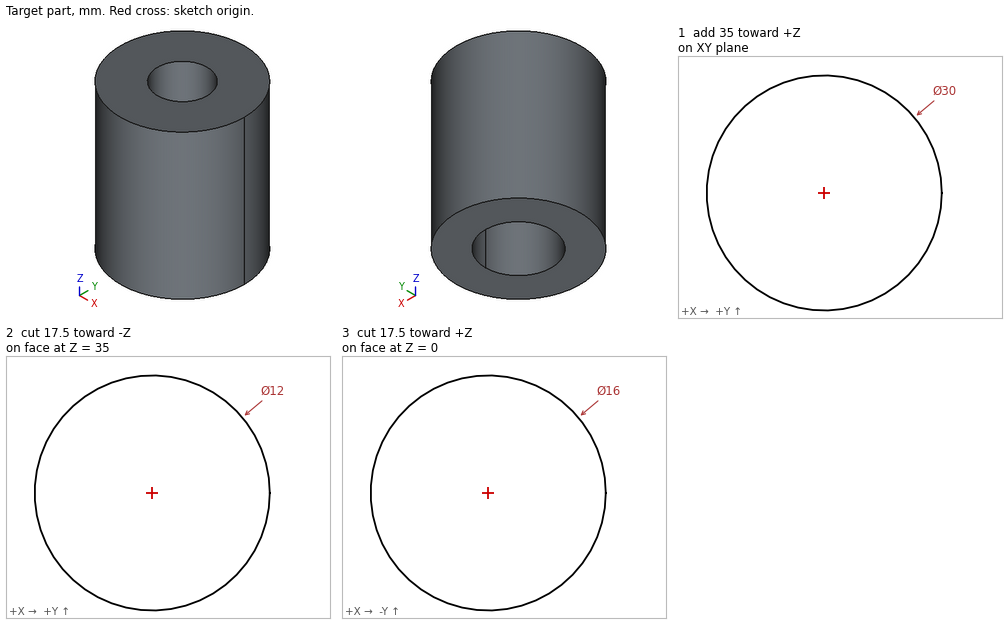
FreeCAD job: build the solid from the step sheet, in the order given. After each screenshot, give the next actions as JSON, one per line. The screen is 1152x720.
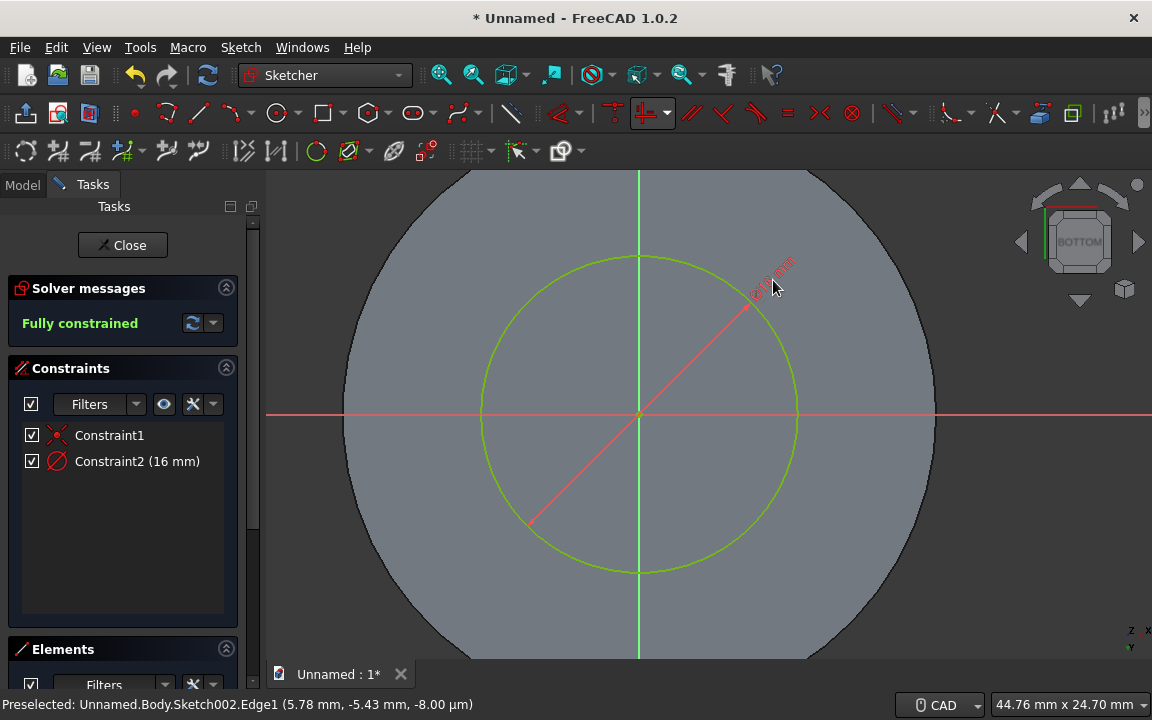
{"action": "left_click", "coordinate": [123, 245]}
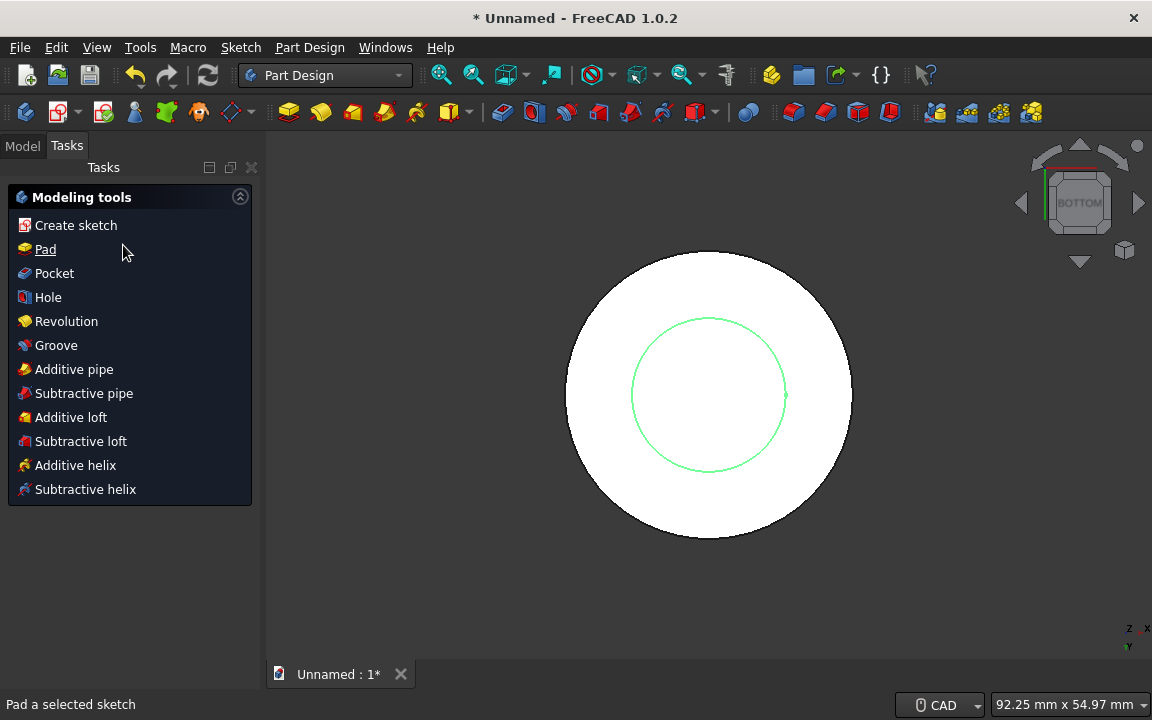
{"action": "left_click", "coordinate": [504, 112]}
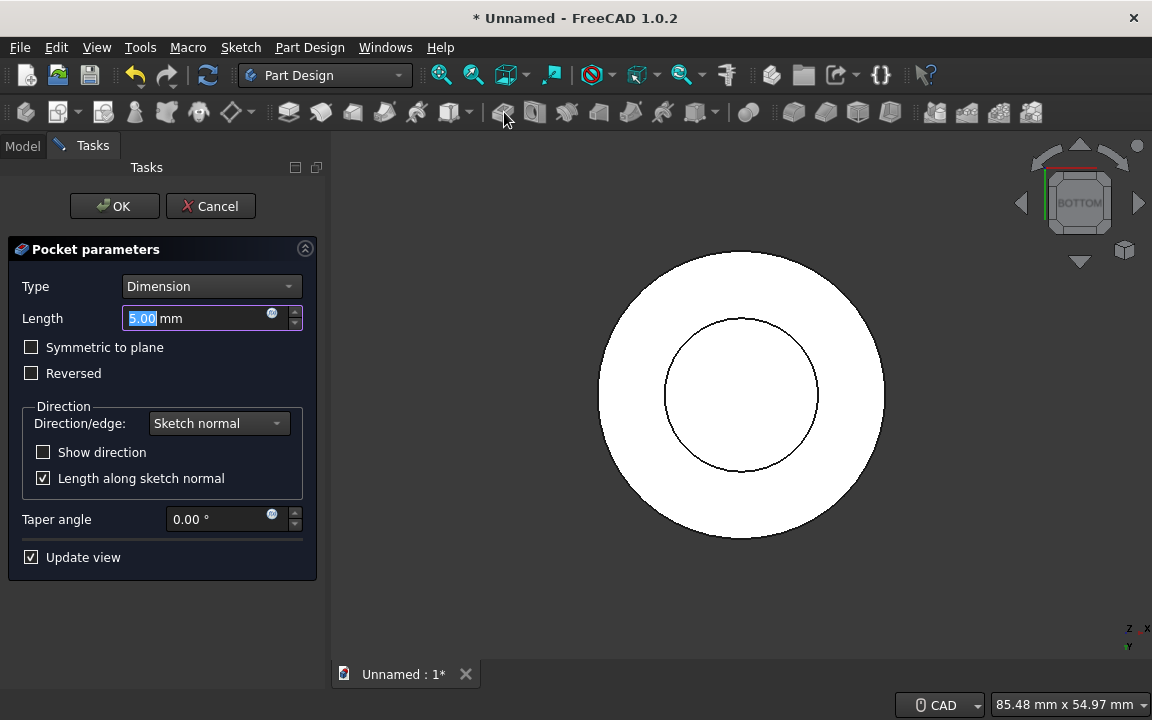
{"action": "type", "text": "17.5"}
{"action": "key", "text": "Tab"}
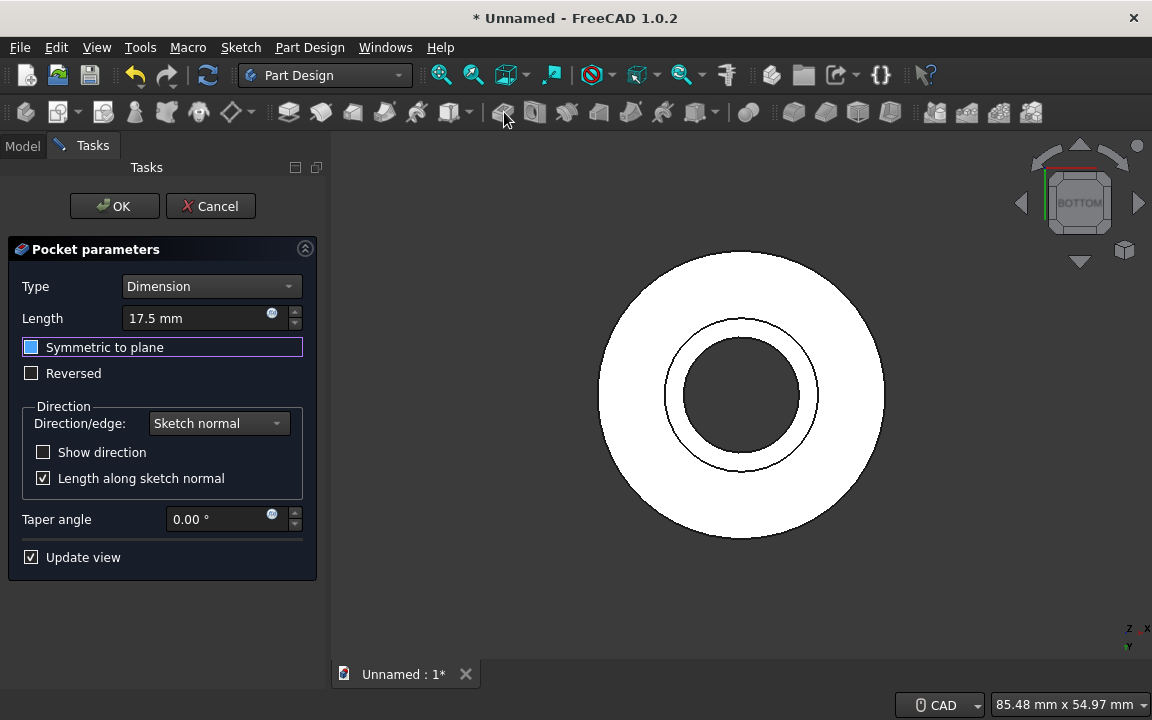
{"action": "left_click", "coordinate": [115, 206]}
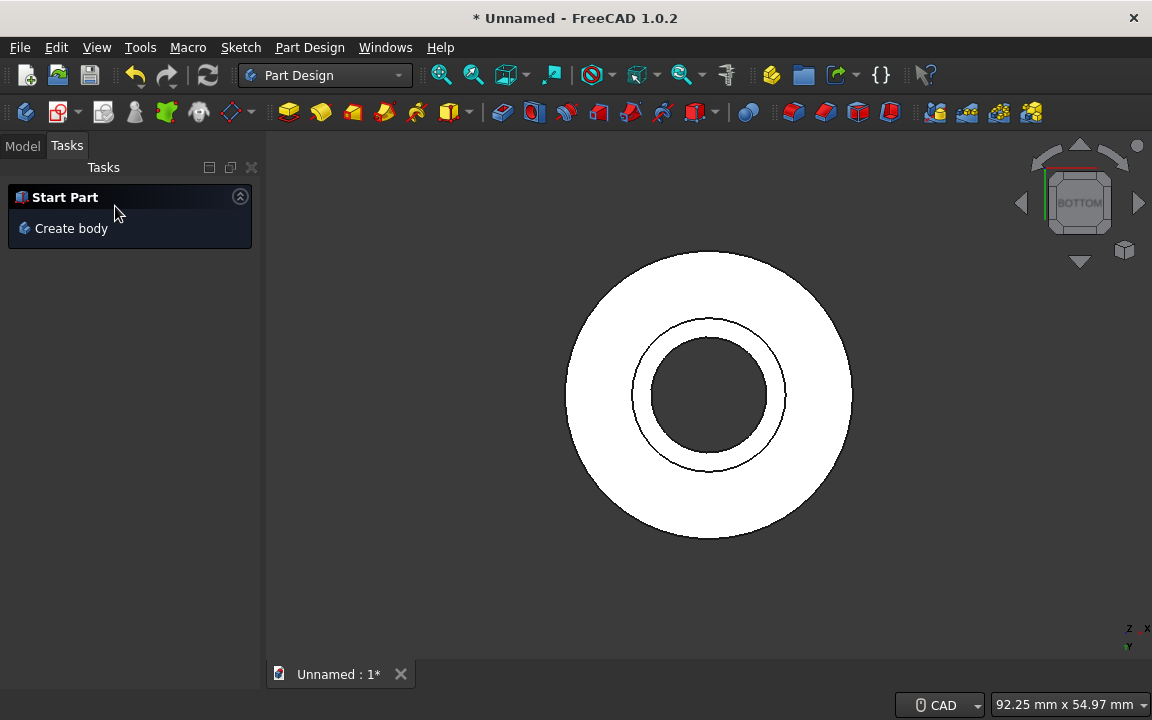
{"action": "key", "text": "0"}